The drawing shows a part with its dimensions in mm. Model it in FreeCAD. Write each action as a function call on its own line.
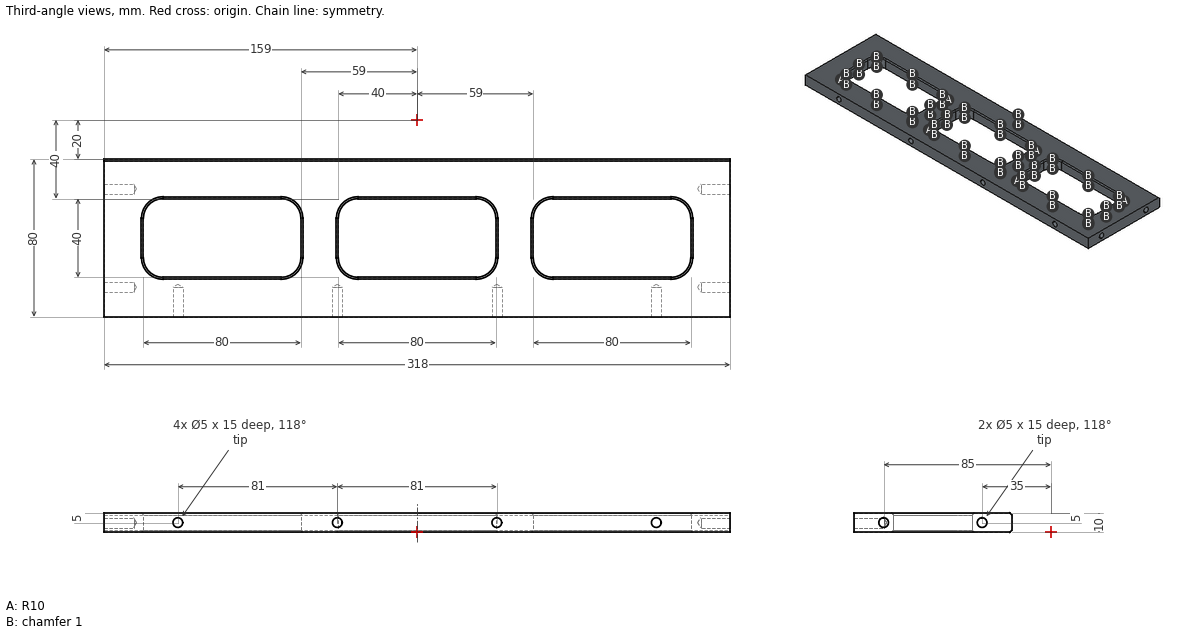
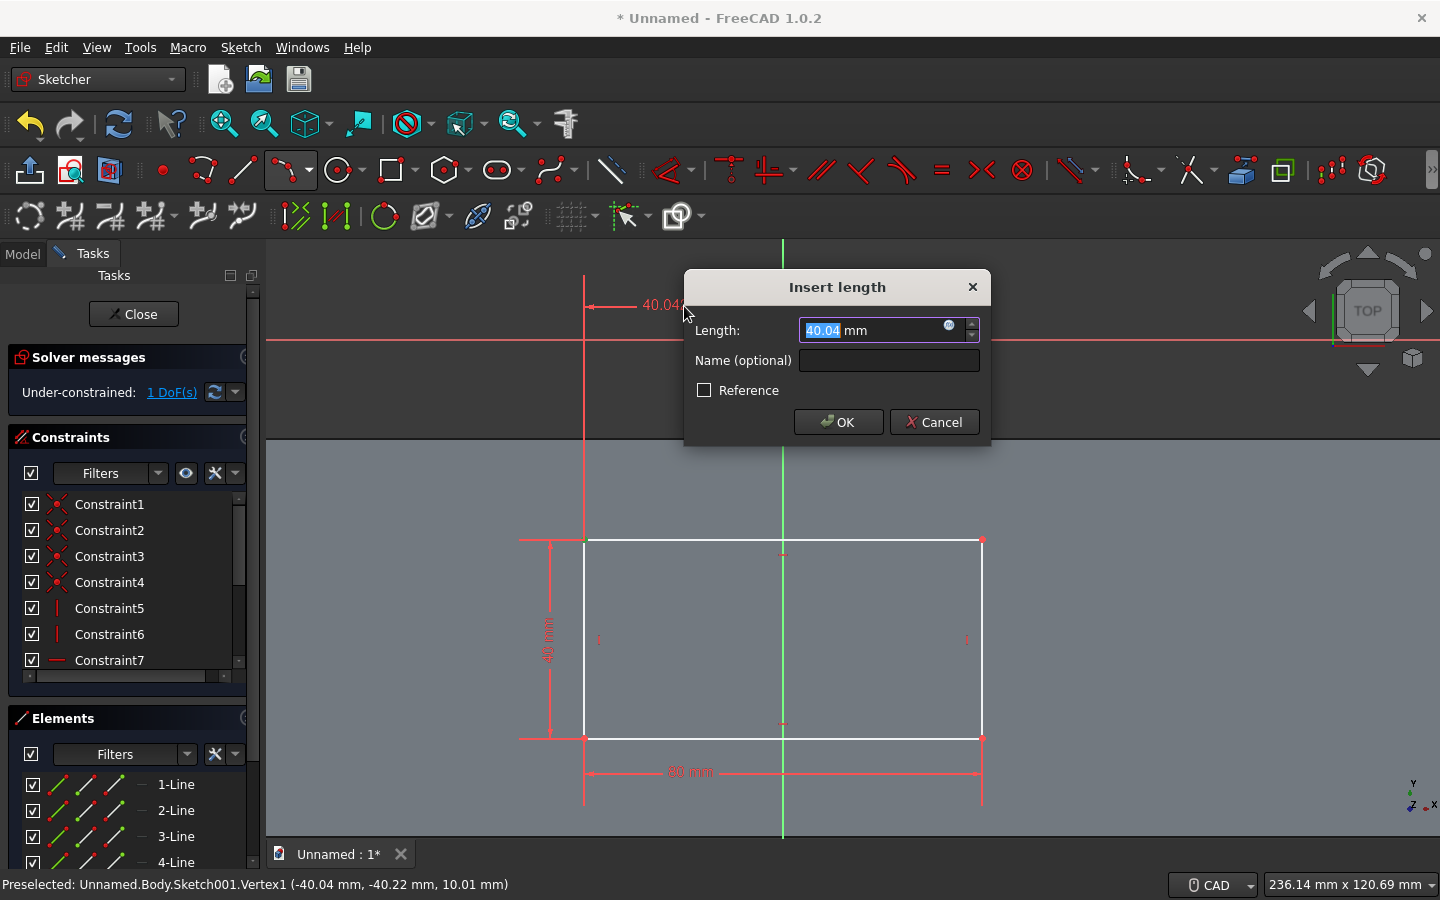
text(40)
key(Return)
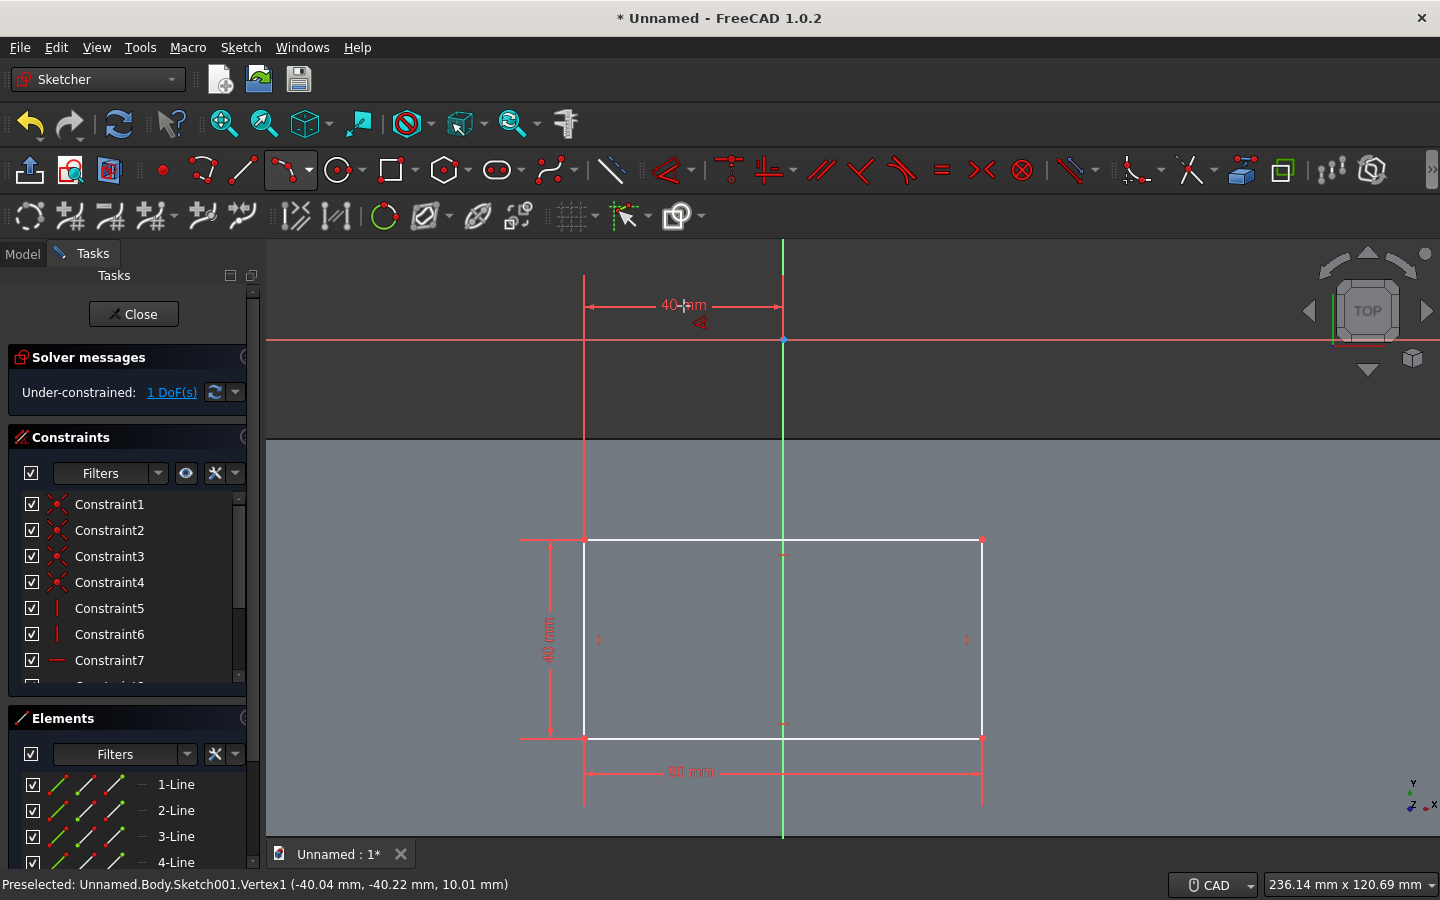
click(584, 540)
click(550, 440)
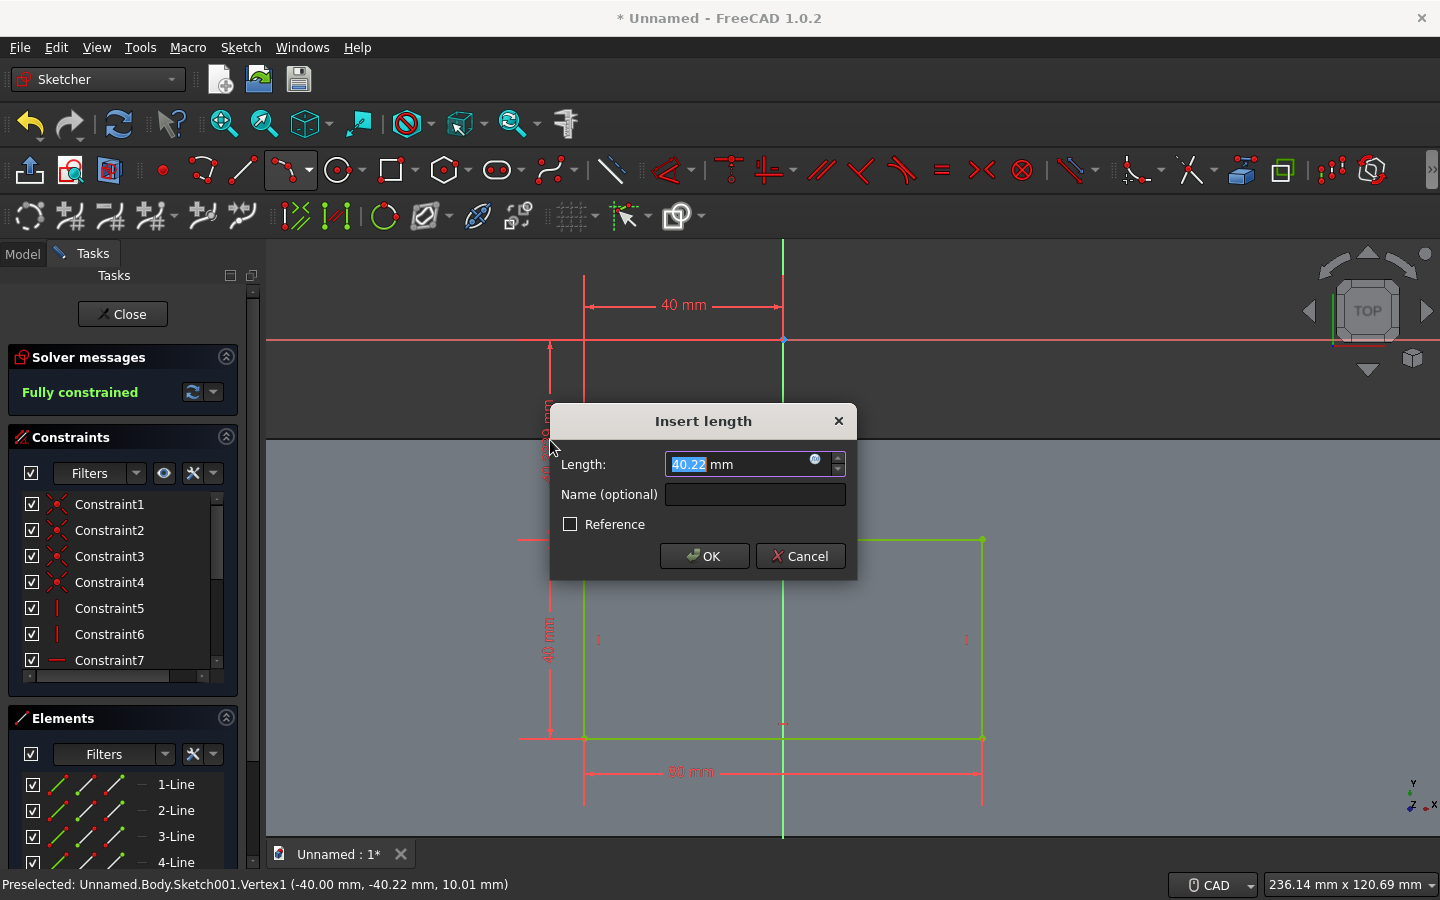
text(40)
key(Return)
key(Escape)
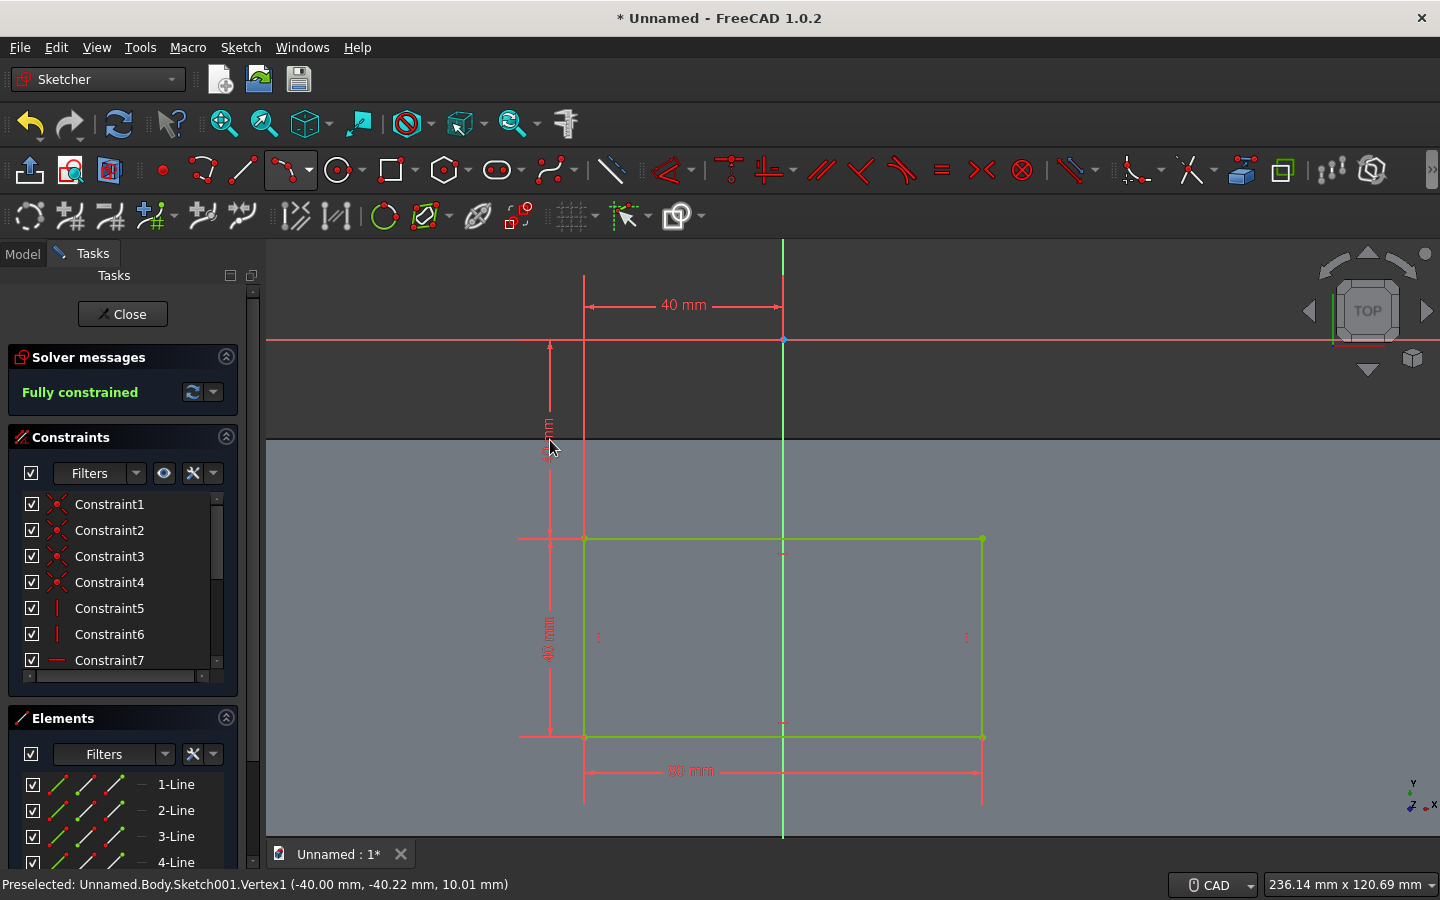
click(123, 314)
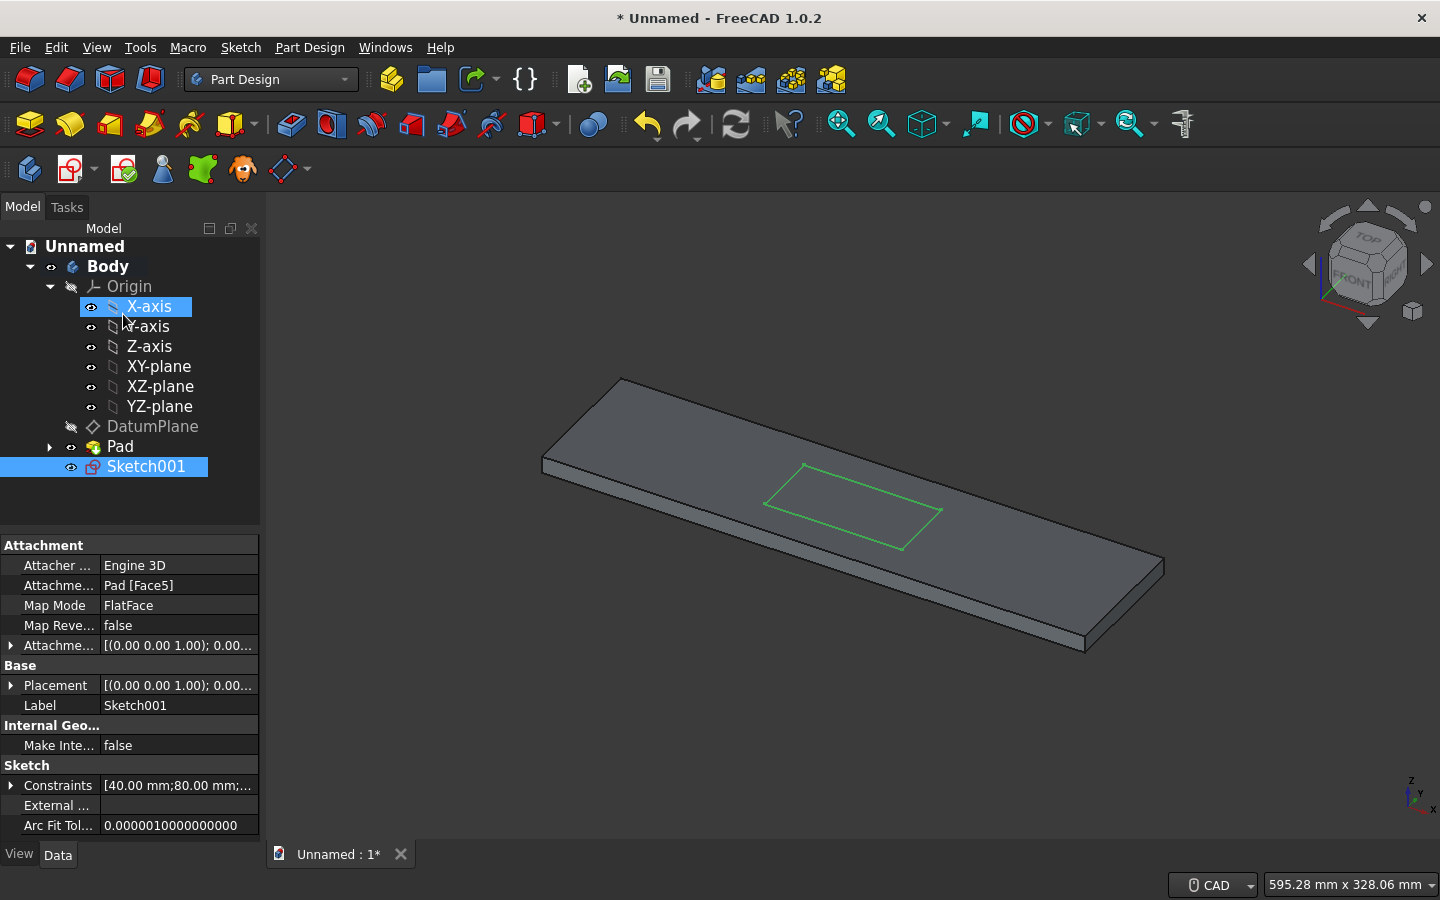
click(292, 124)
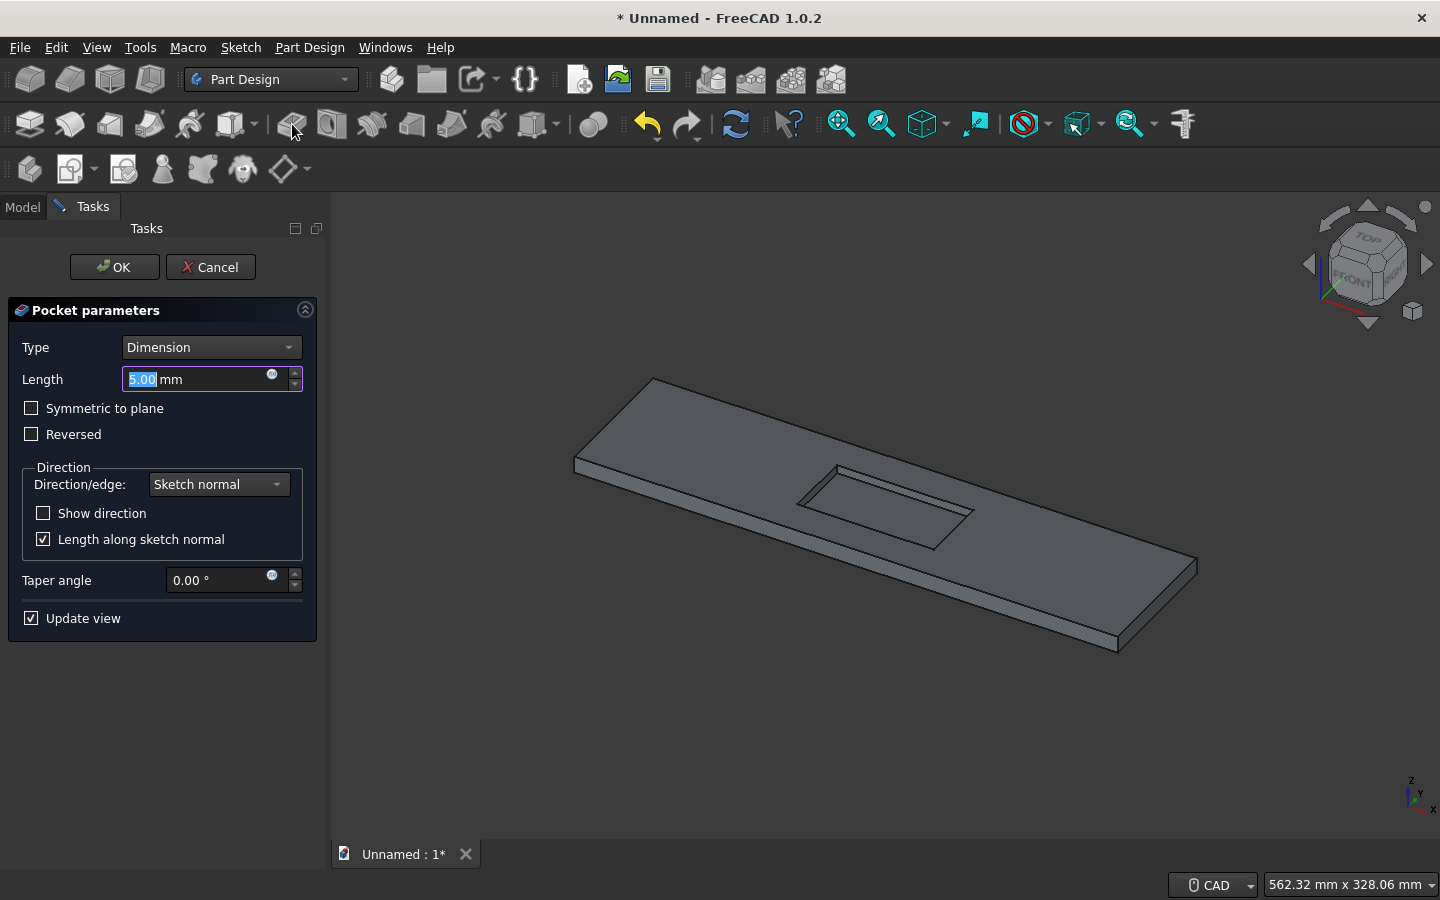
click(212, 348)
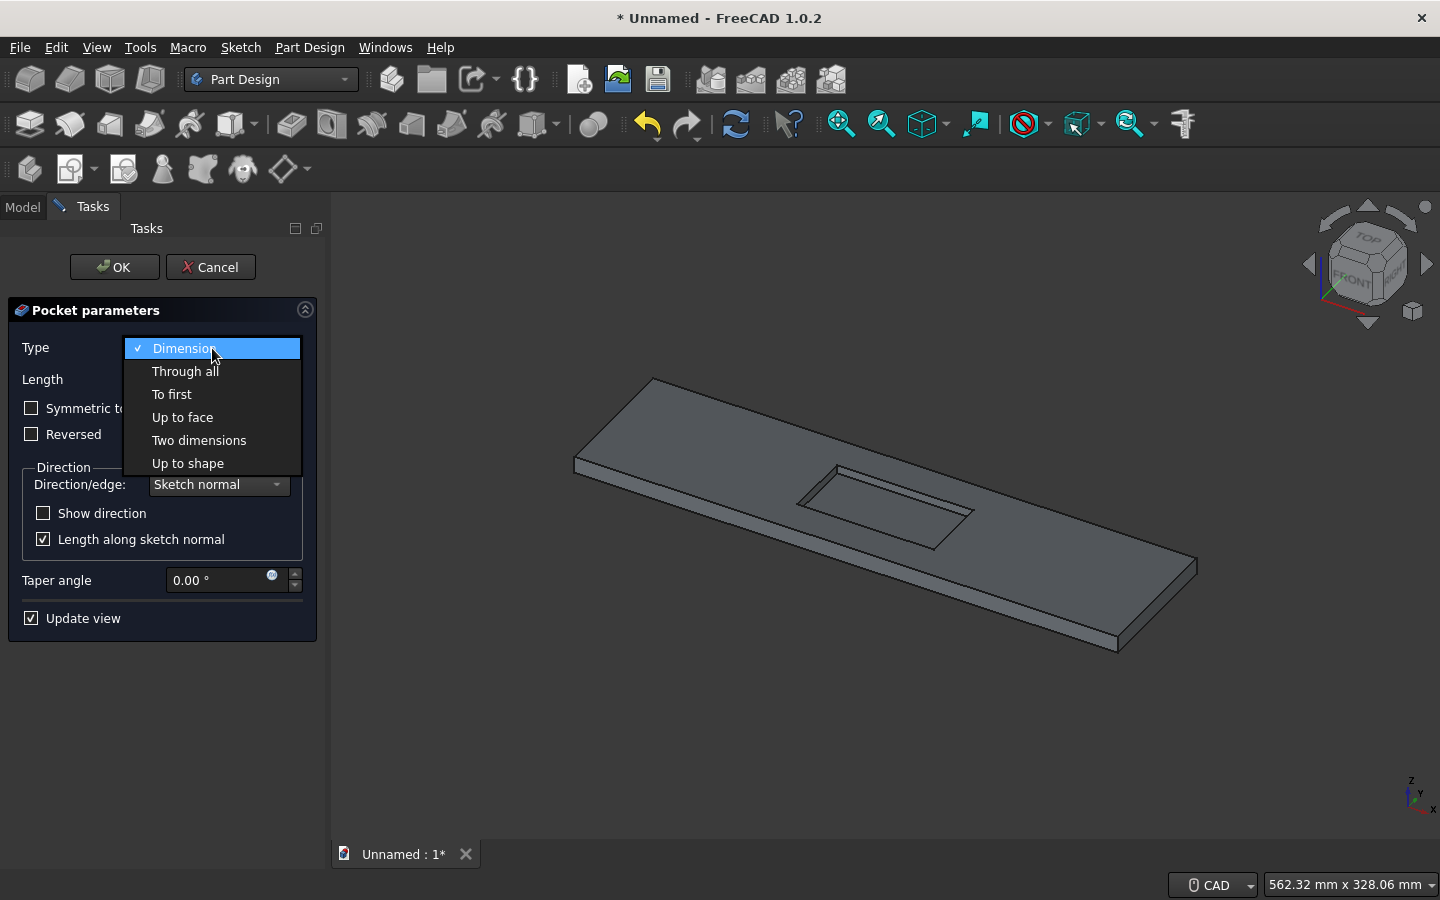
click(212, 372)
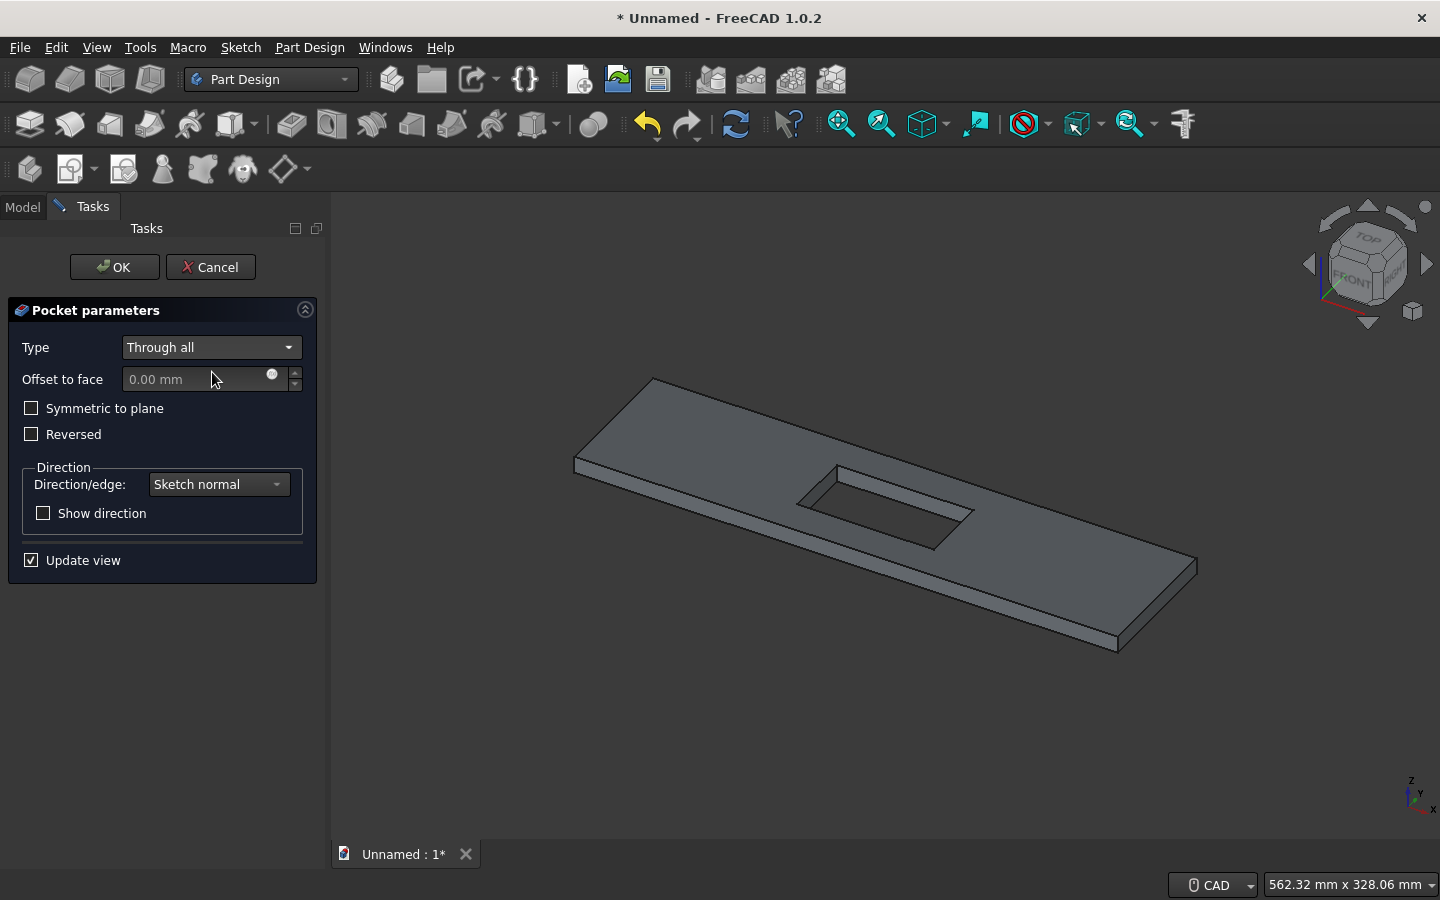
click(115, 267)